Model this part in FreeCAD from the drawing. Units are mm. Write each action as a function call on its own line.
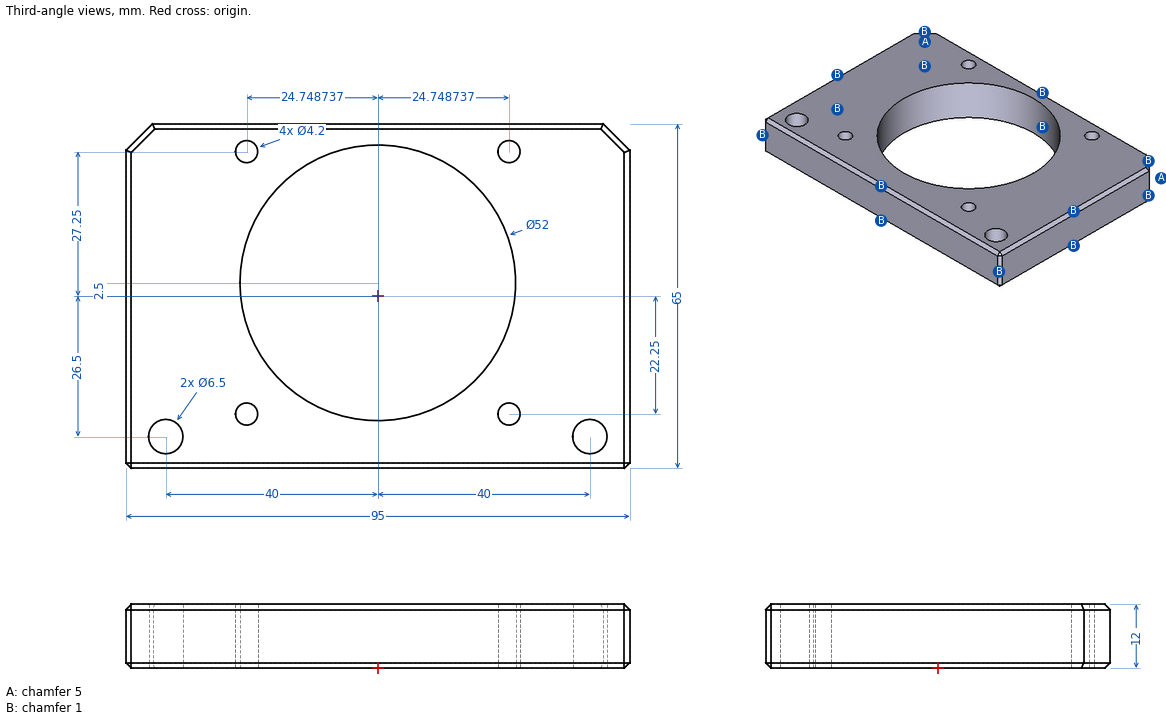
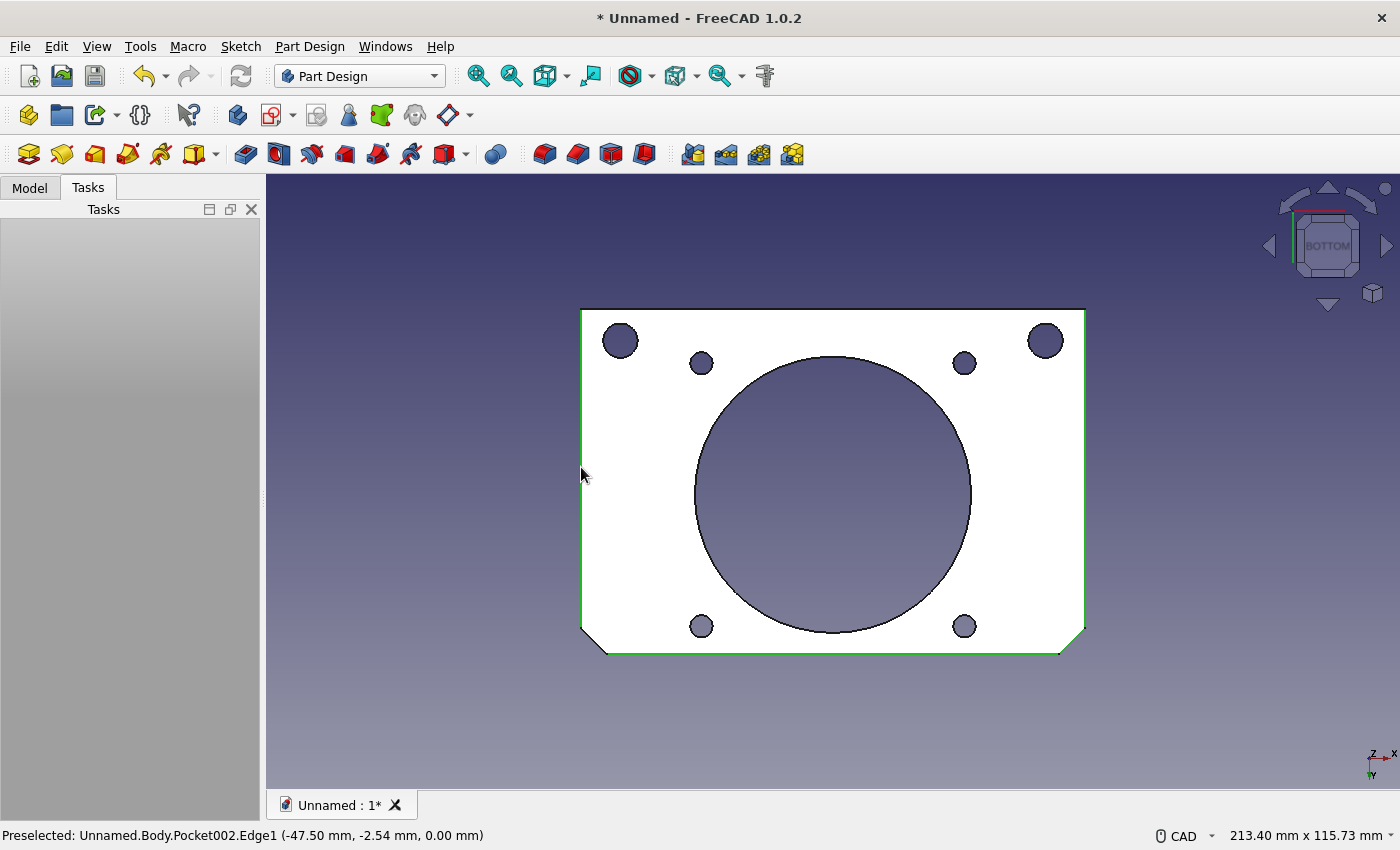
click(594, 640, ctrl)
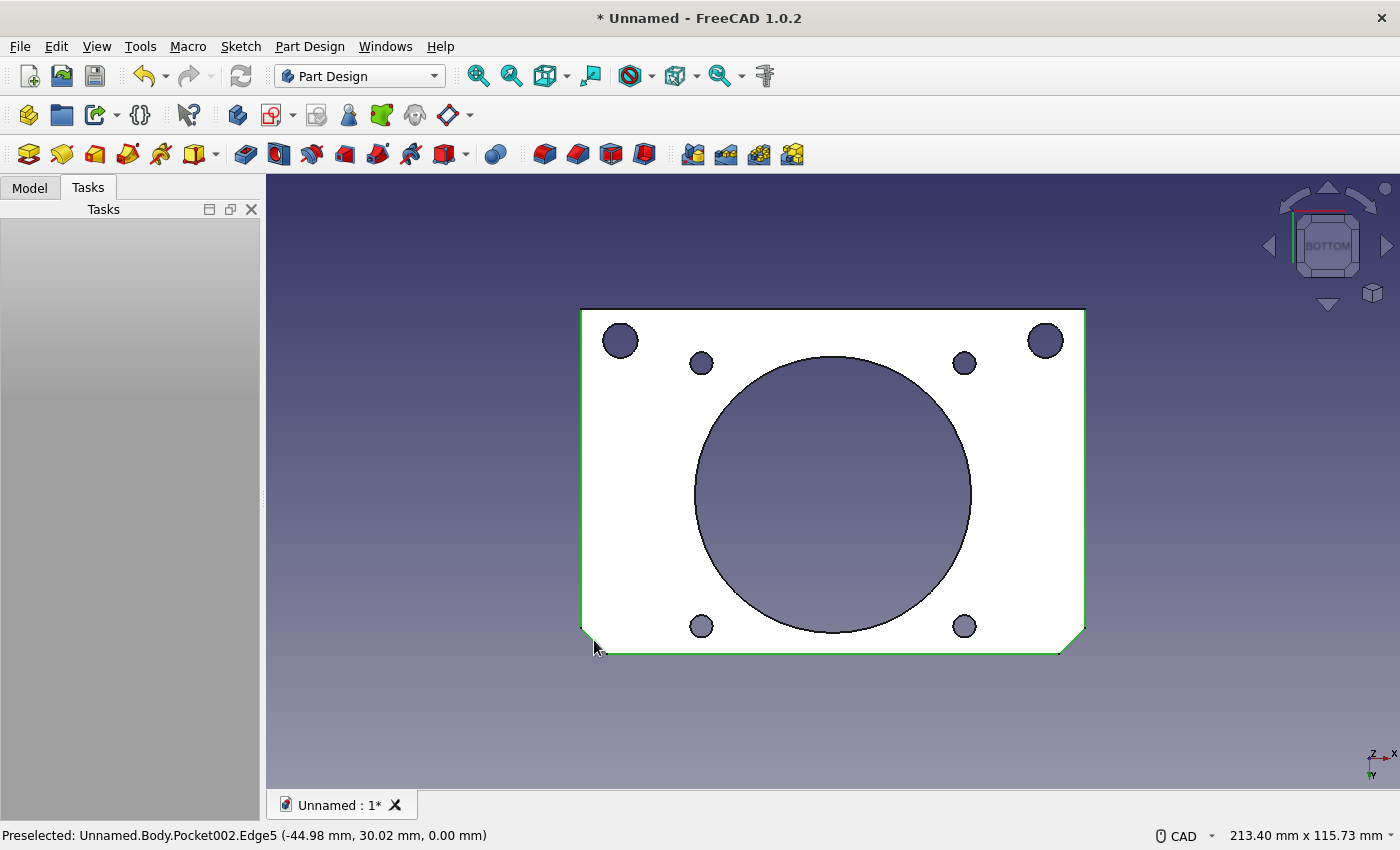
click(578, 154)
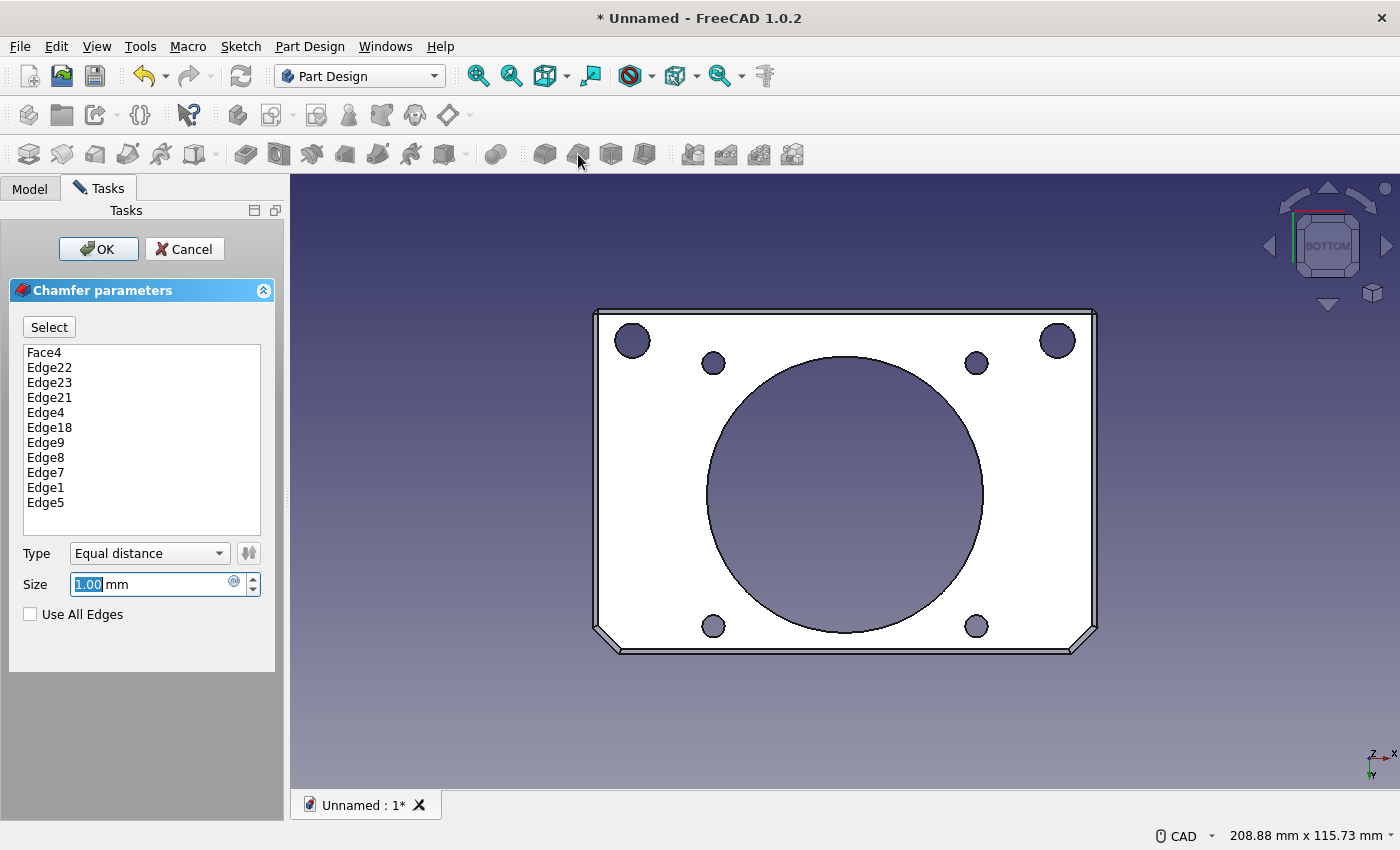
text(1)
key(Tab)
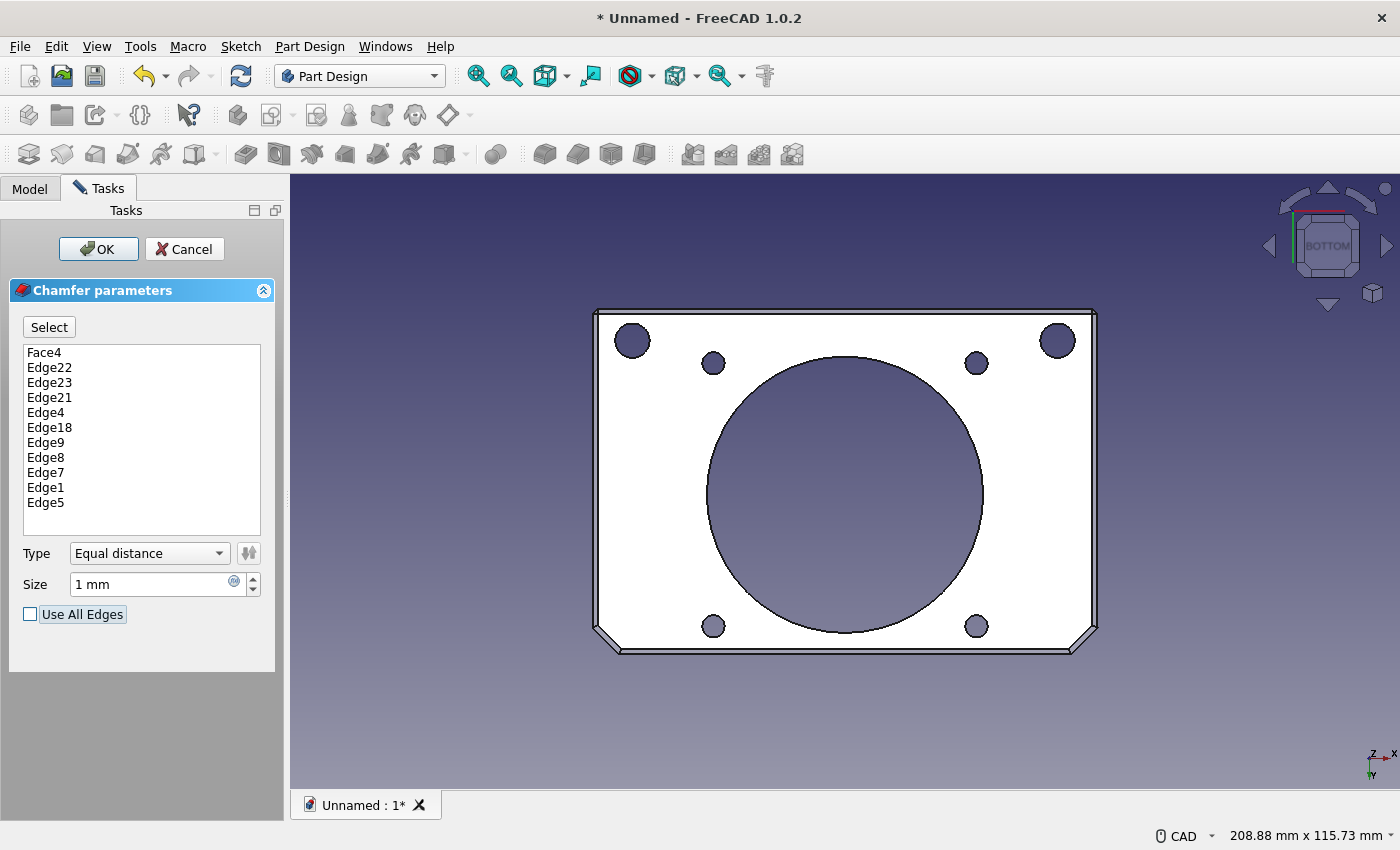
click(99, 249)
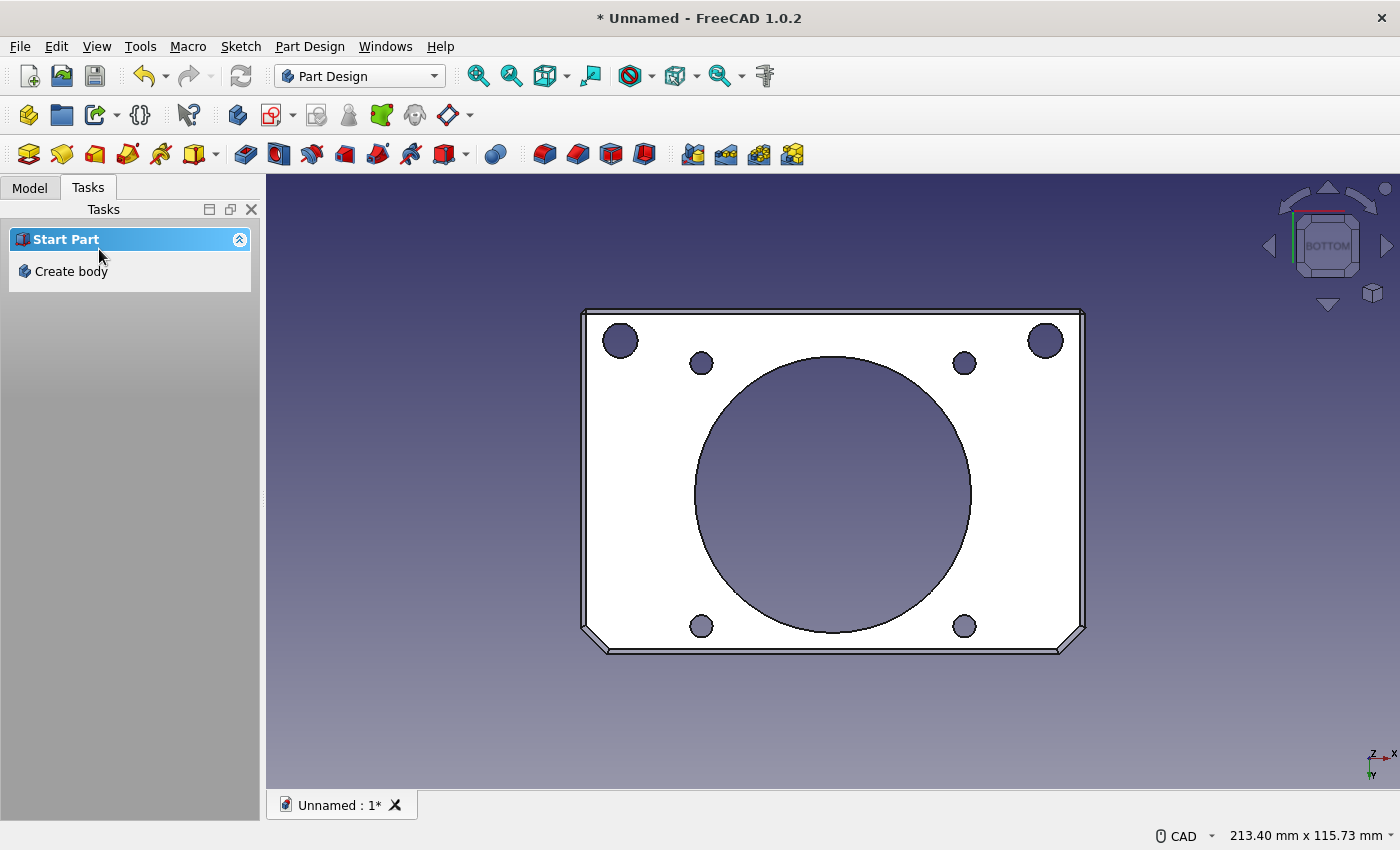
key(0)